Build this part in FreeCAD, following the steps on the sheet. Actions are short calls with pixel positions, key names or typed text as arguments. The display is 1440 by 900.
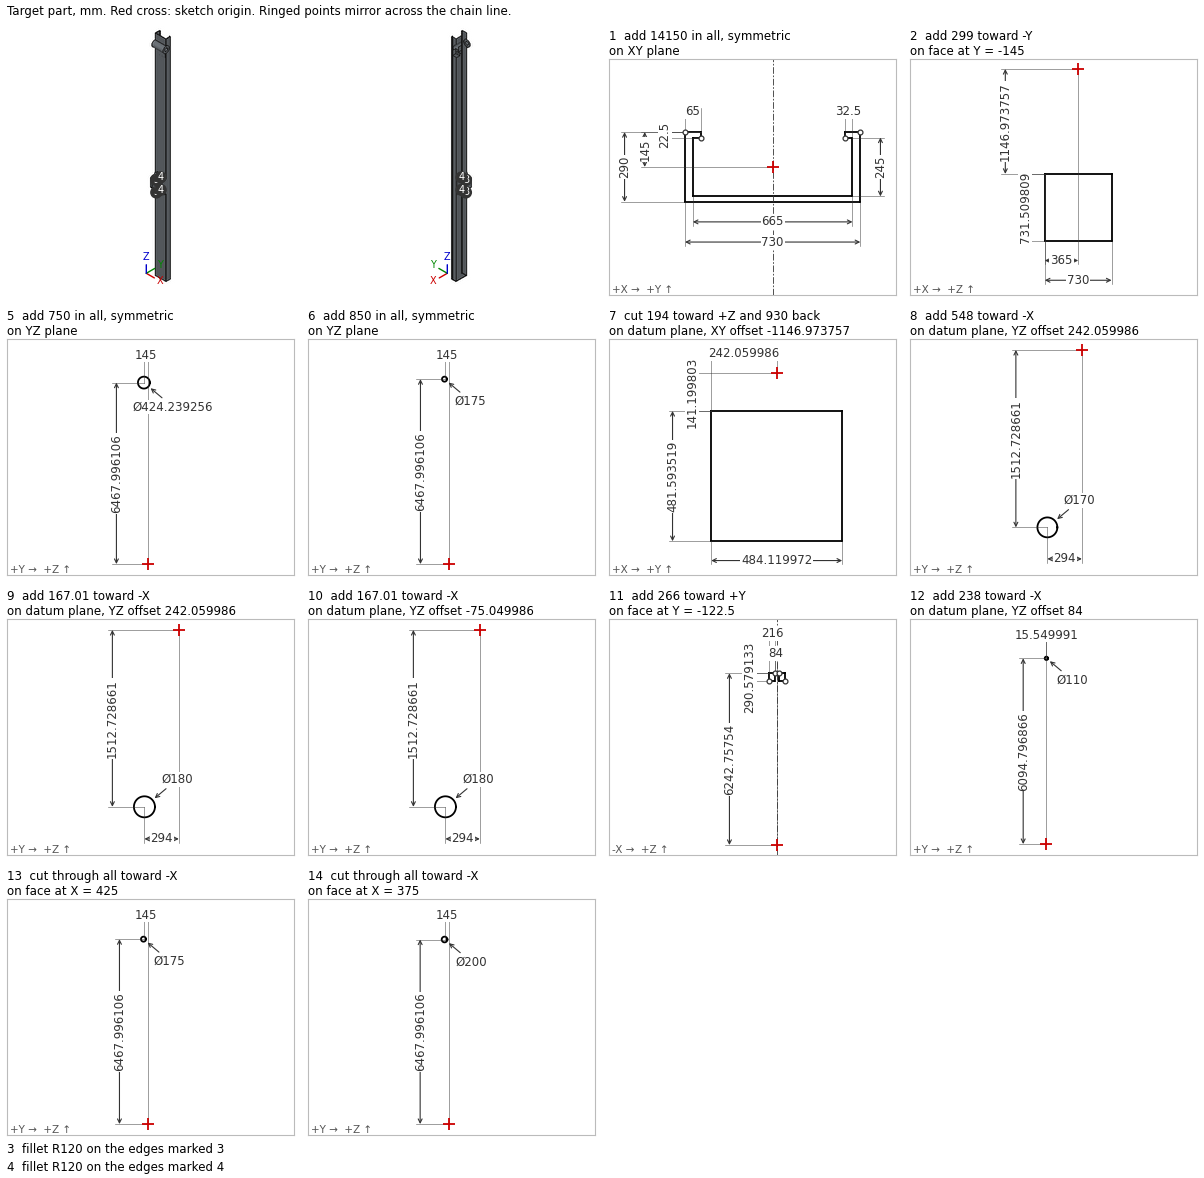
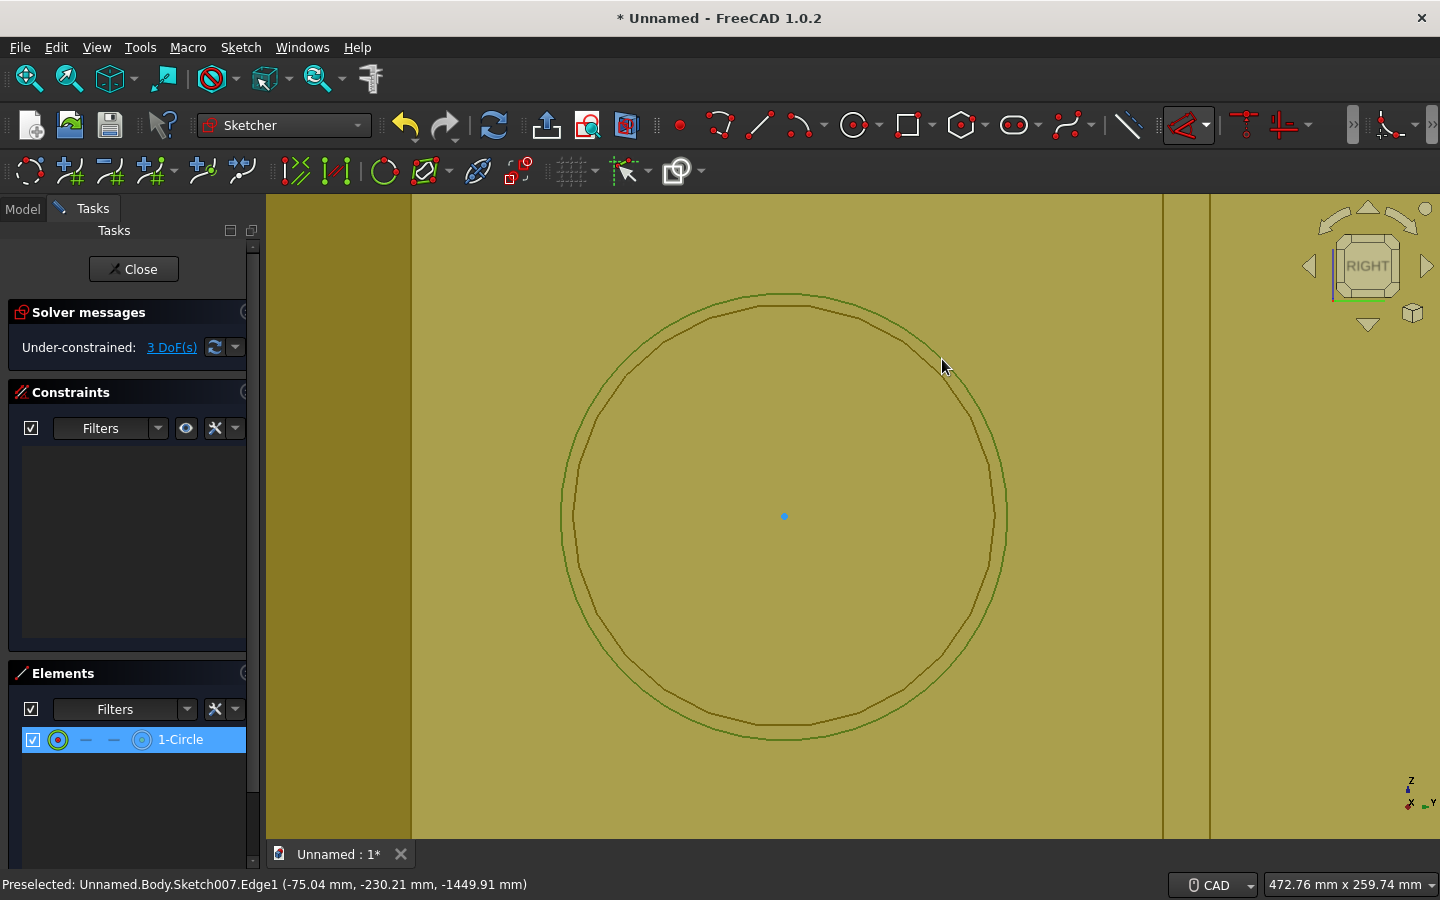
key(k)
key(o)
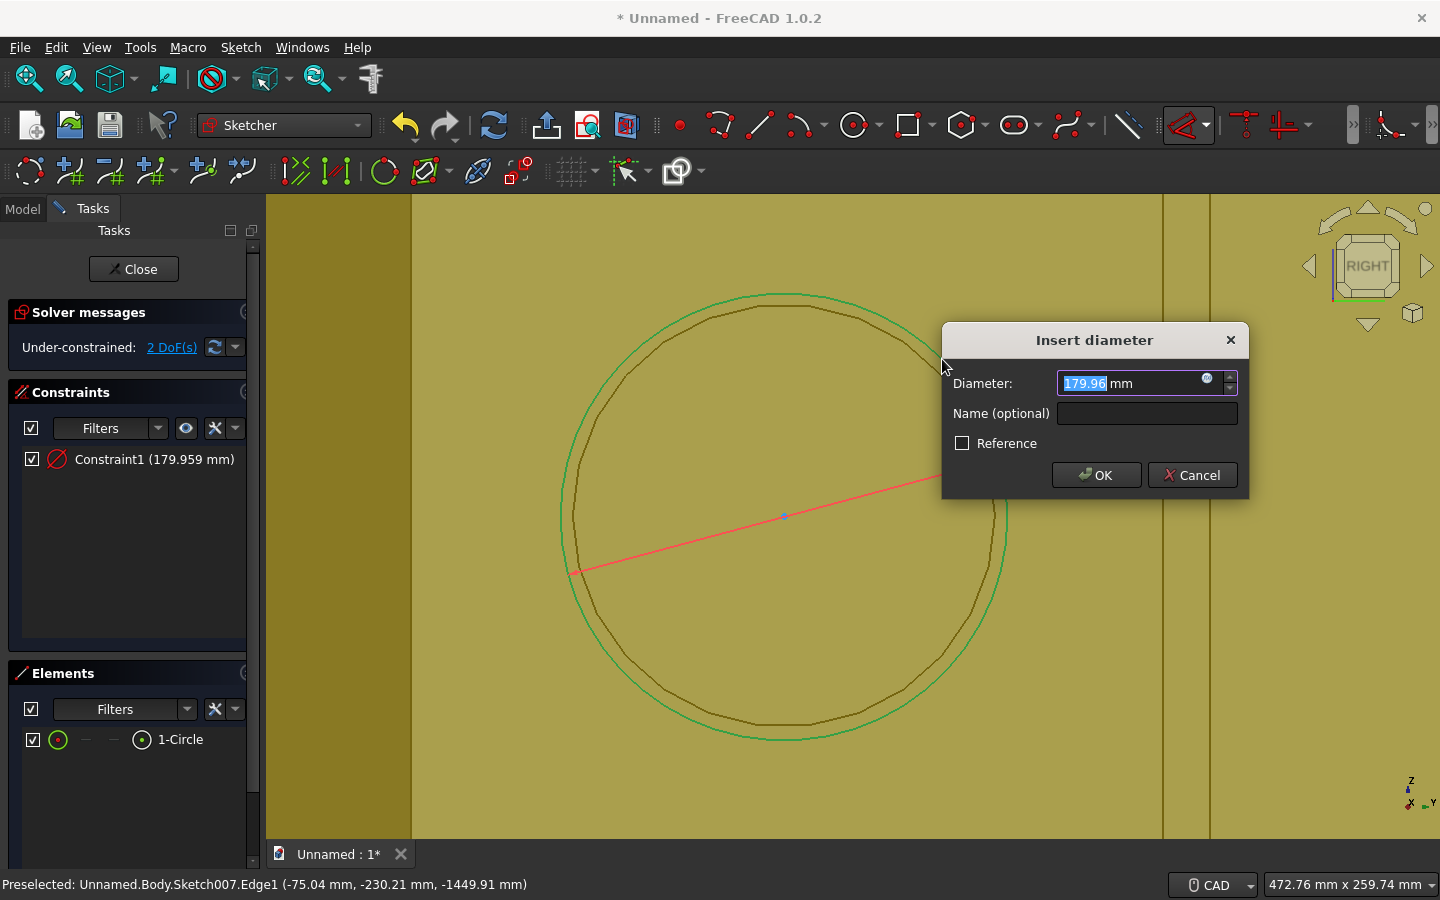
text(180)
key(Return)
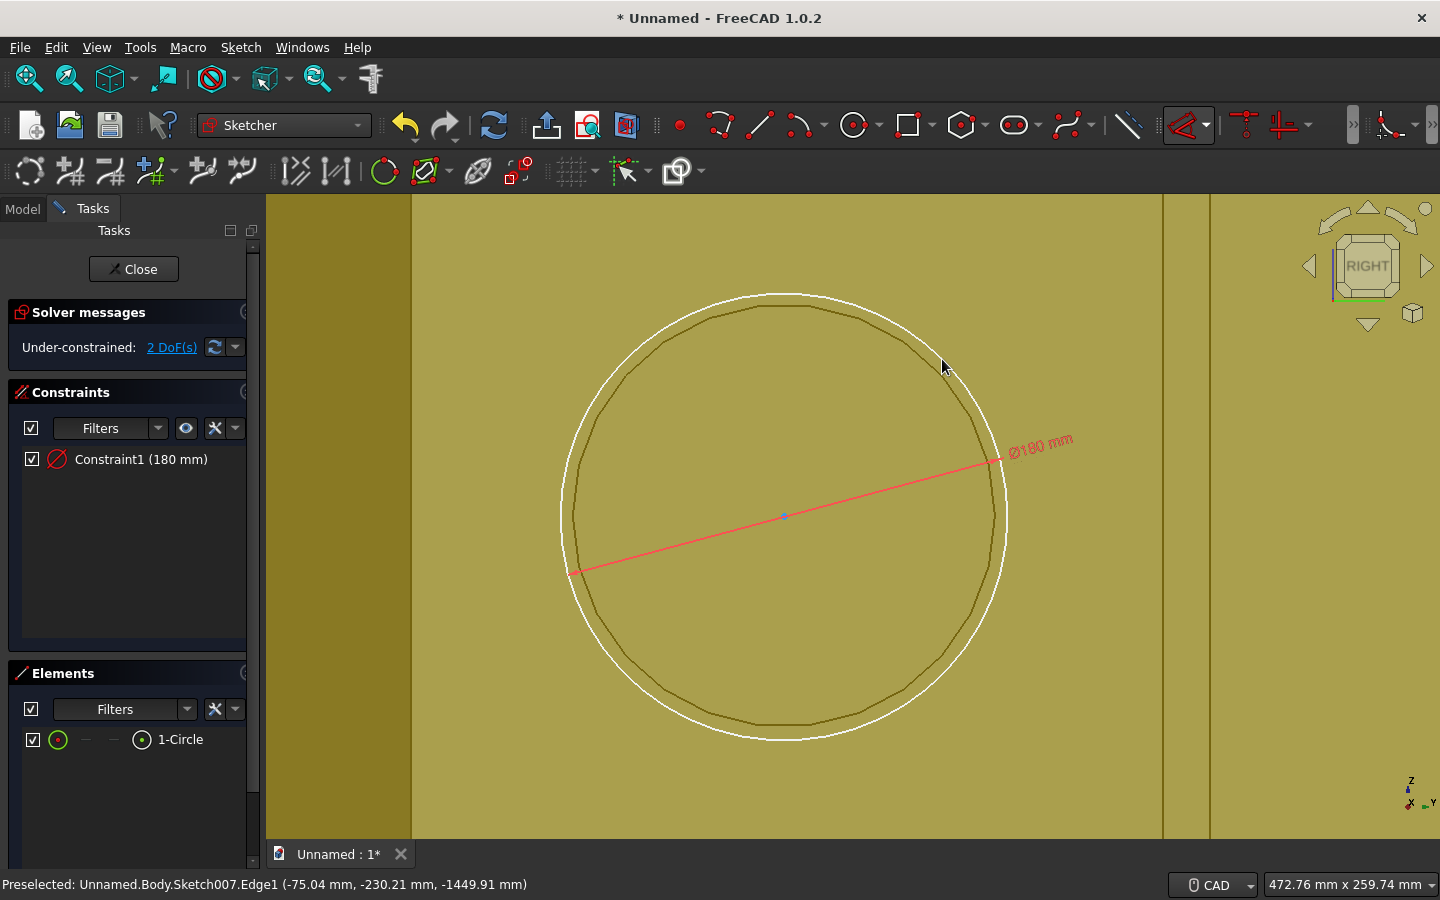
click(784, 517)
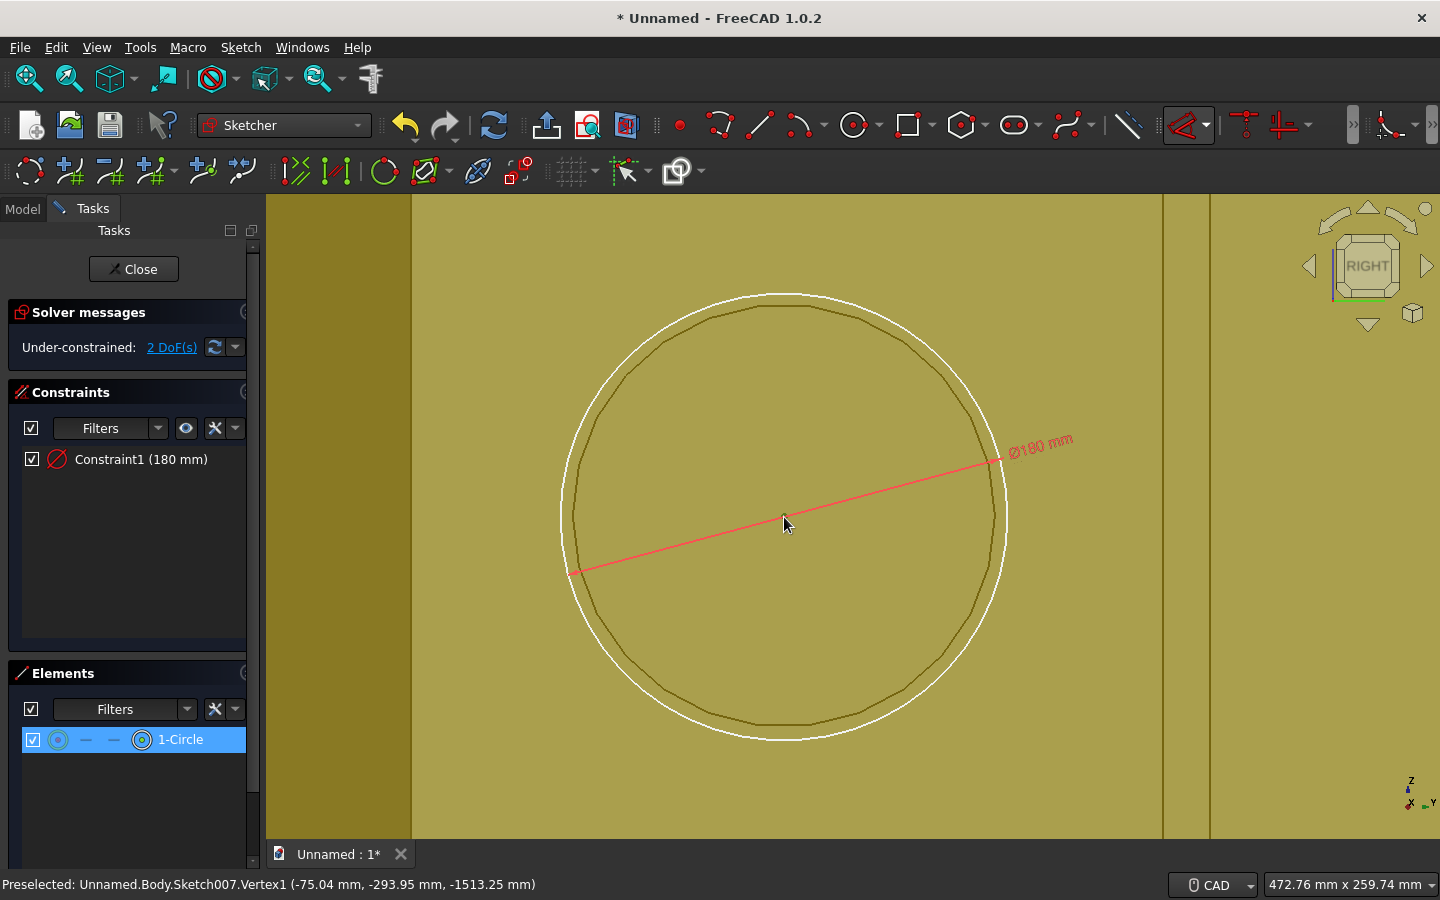
key(l)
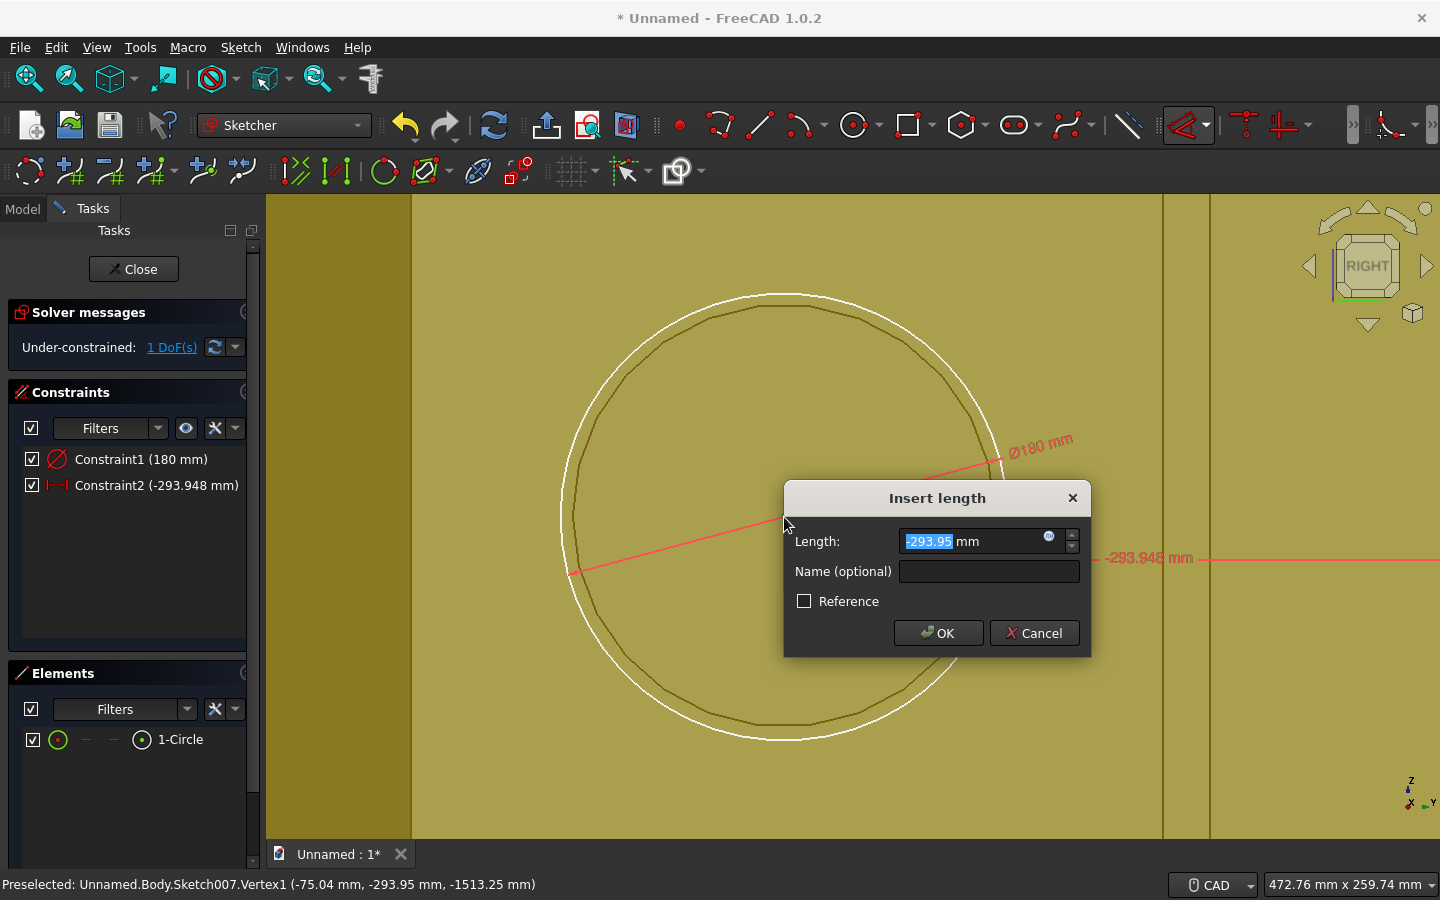
text(-294)
key(Return)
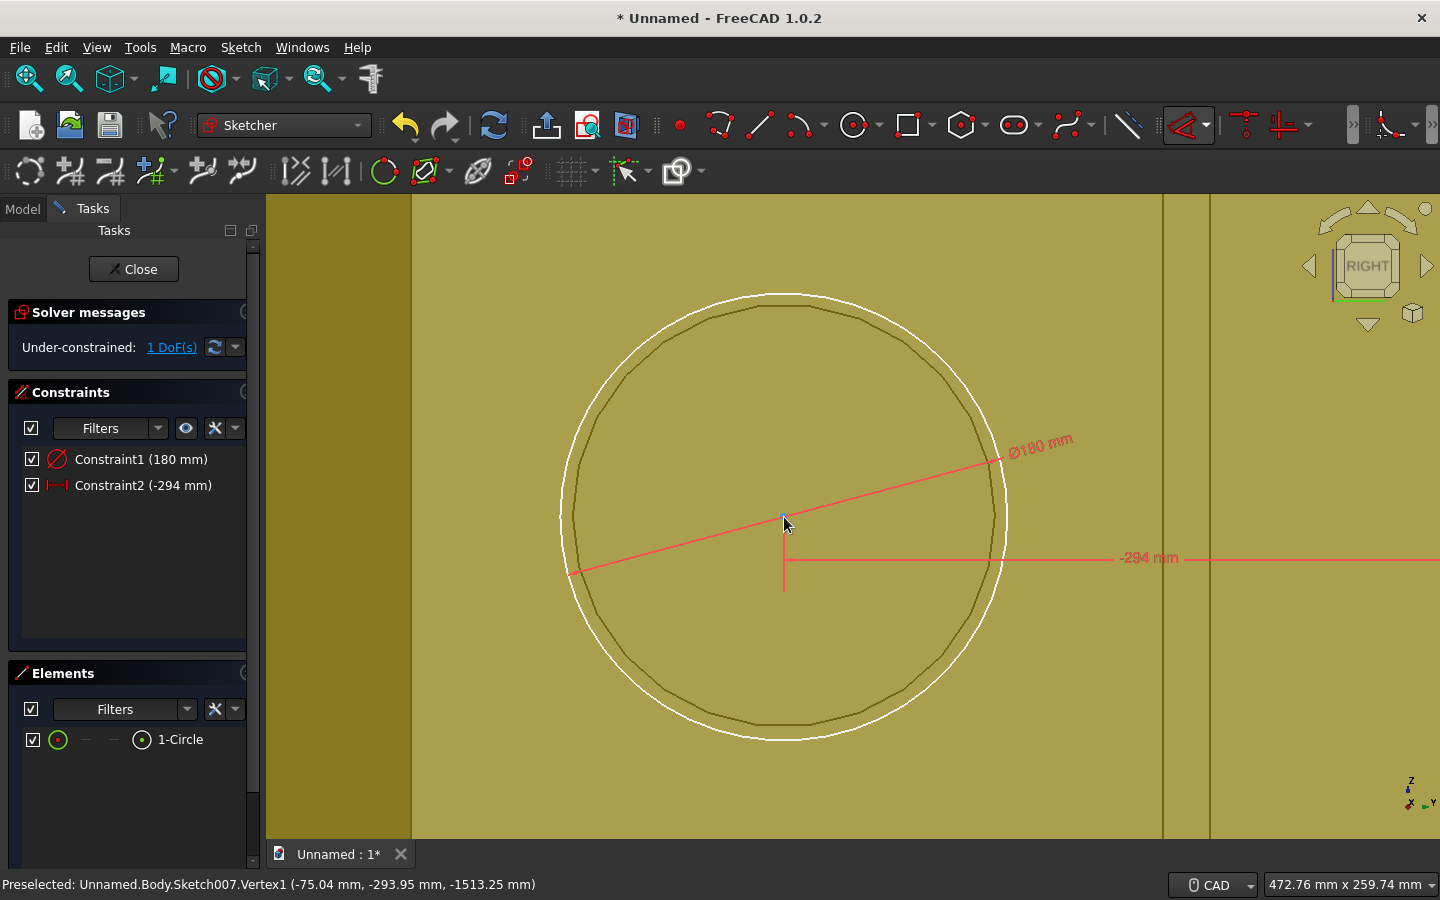
click(784, 517)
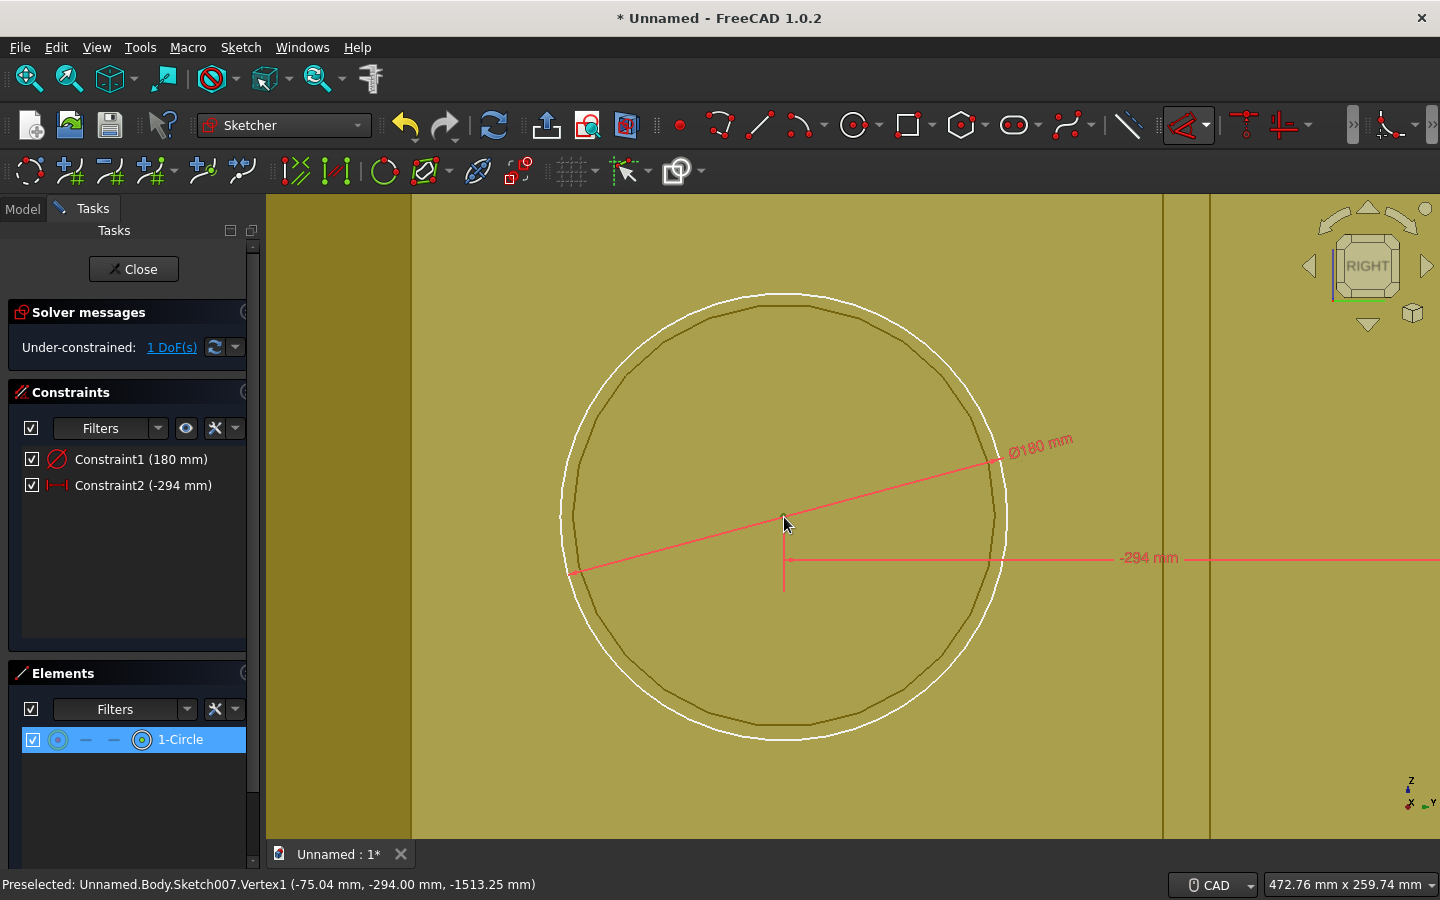
key(i)